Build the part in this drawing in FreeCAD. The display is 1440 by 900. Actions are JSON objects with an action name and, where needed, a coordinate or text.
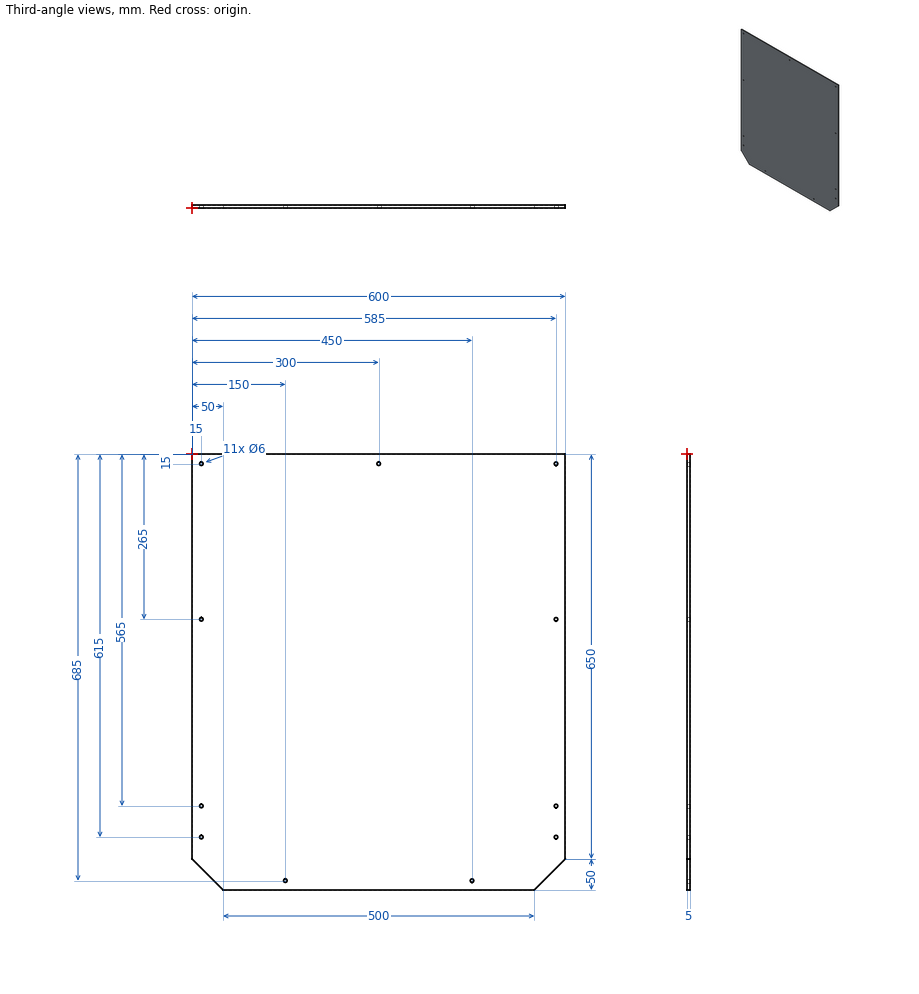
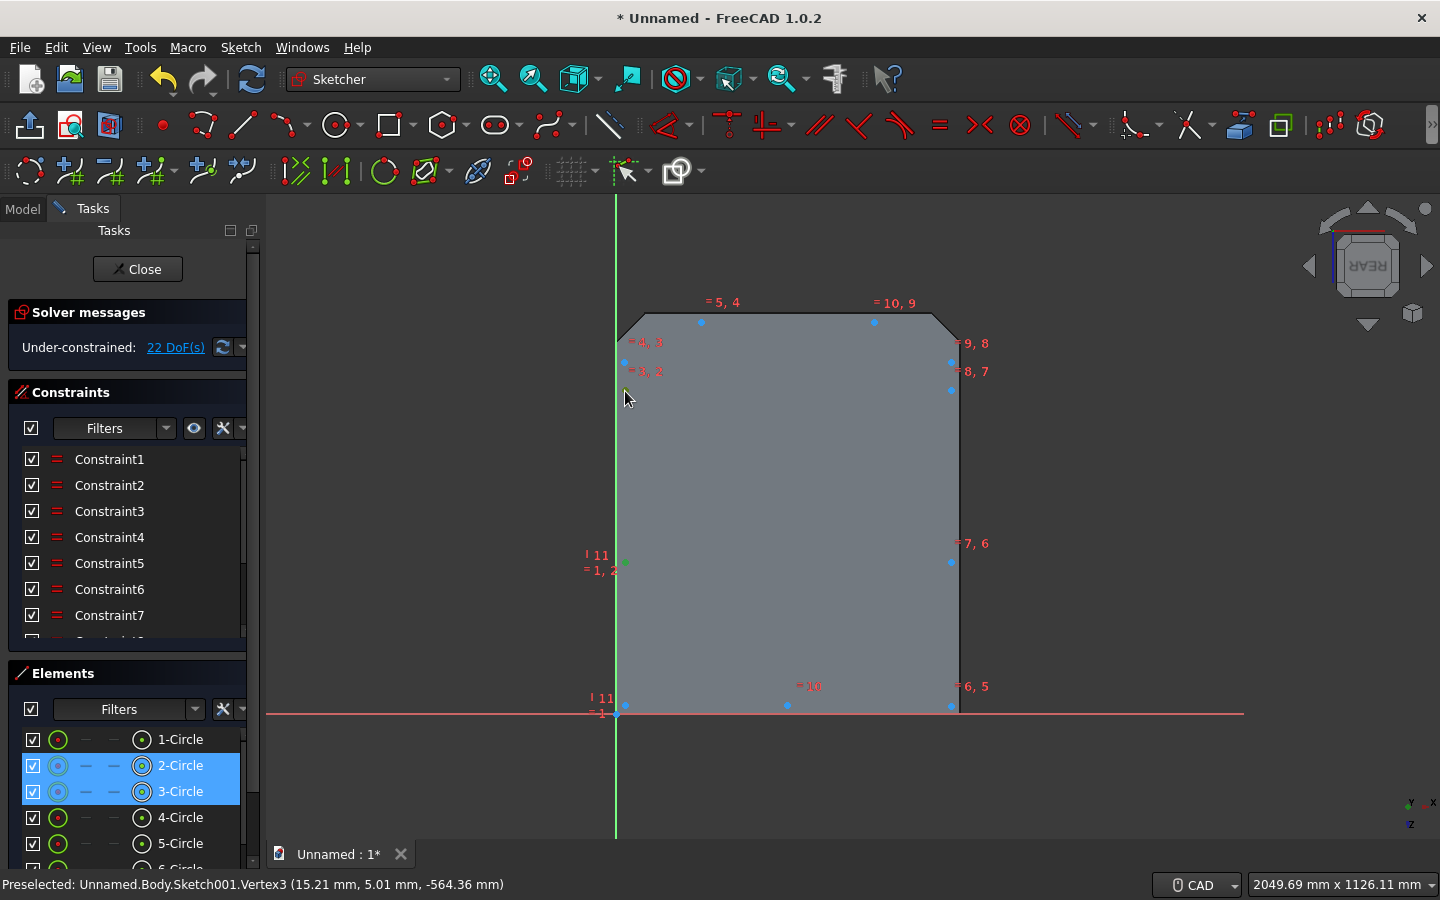
{"action": "key", "text": "v"}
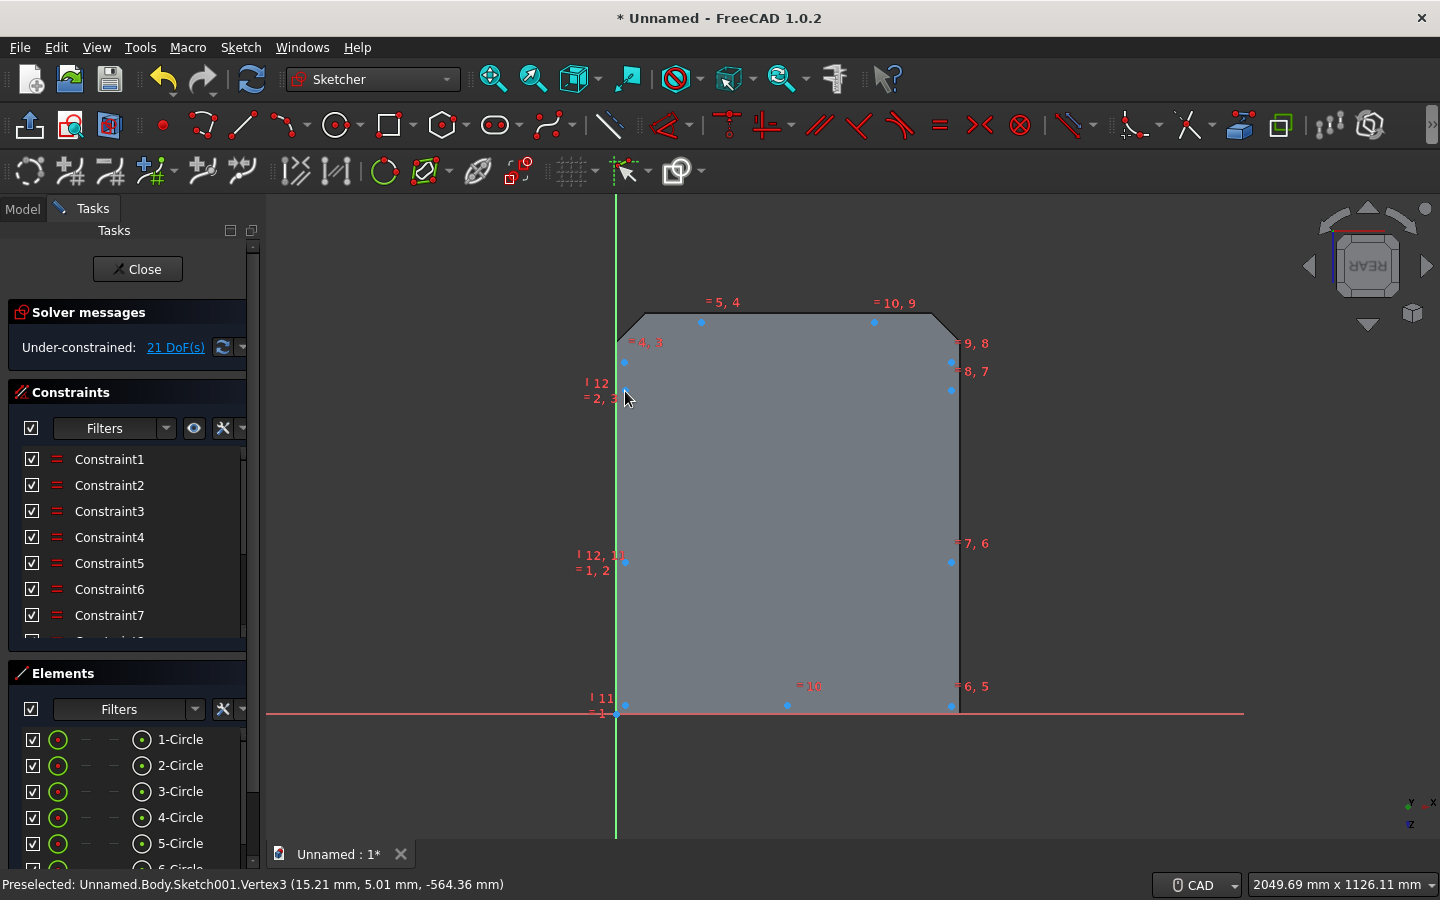
{"action": "left_click", "coordinate": [625, 391]}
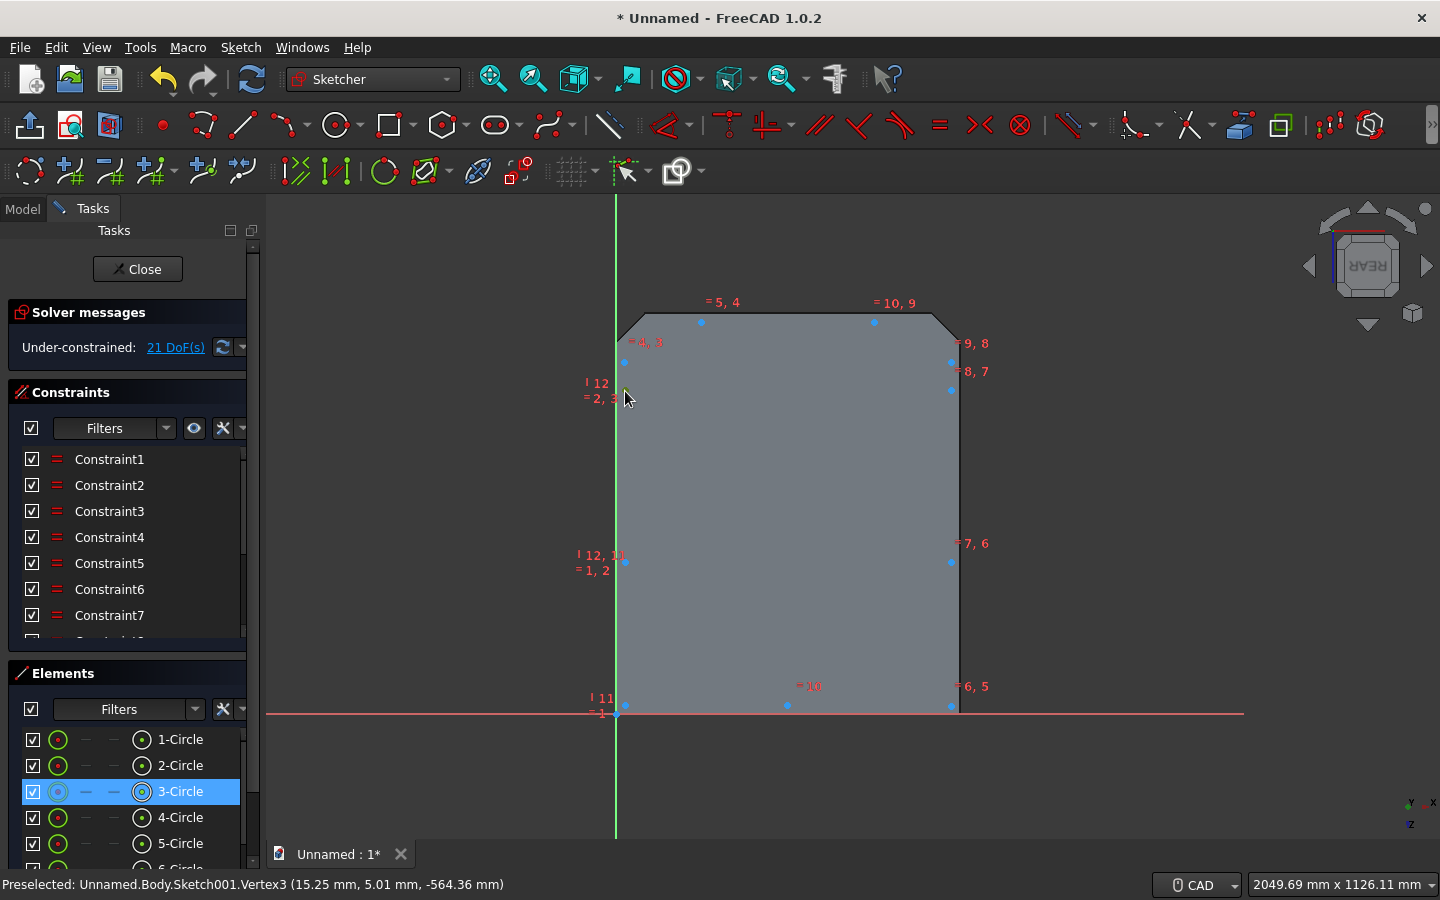
{"action": "left_click", "coordinate": [625, 362]}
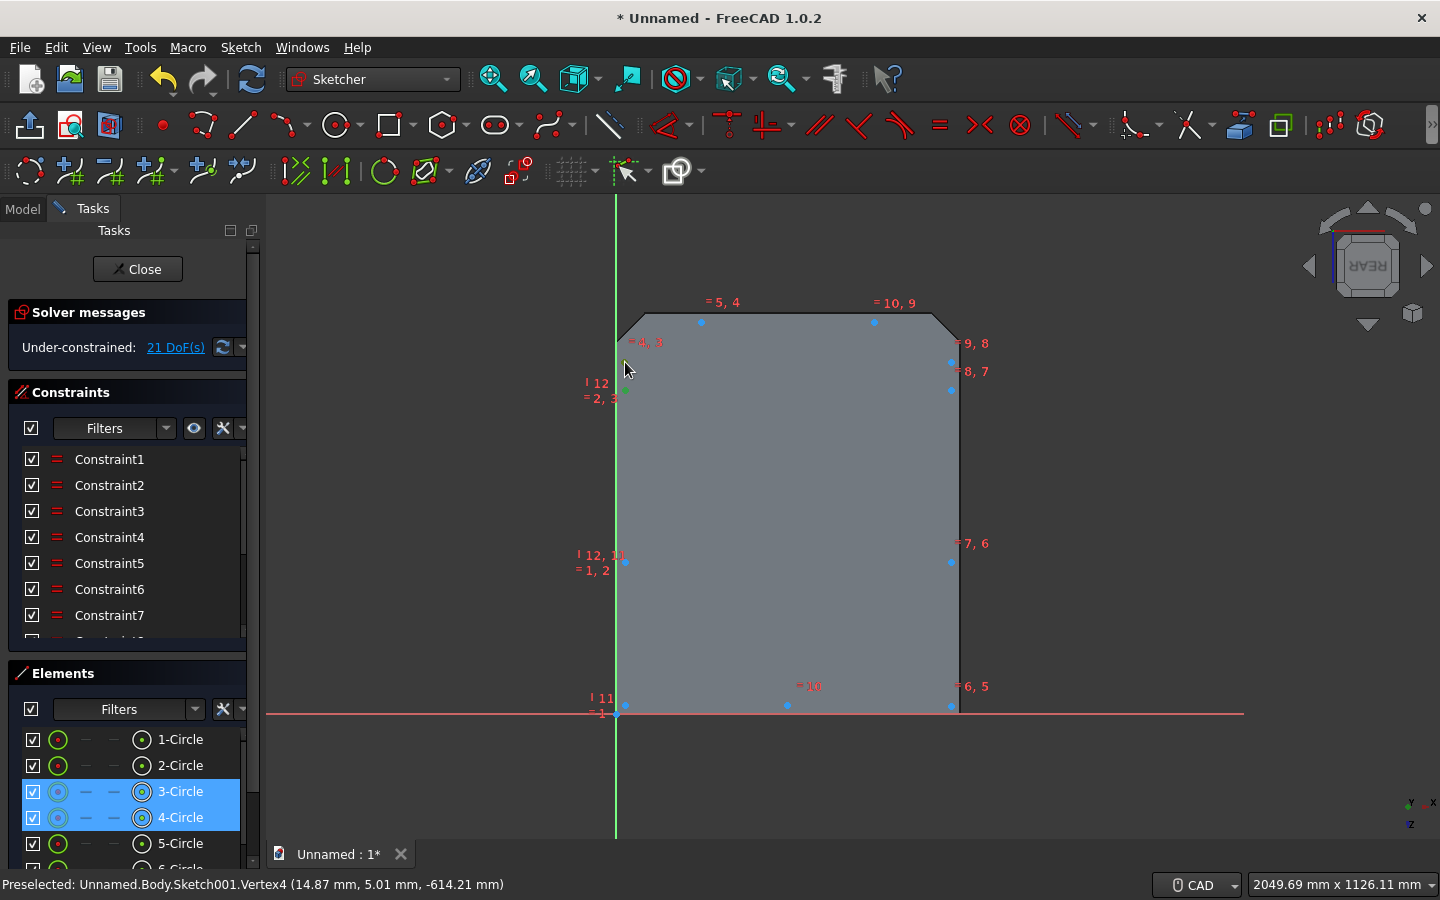
{"action": "key", "text": "v"}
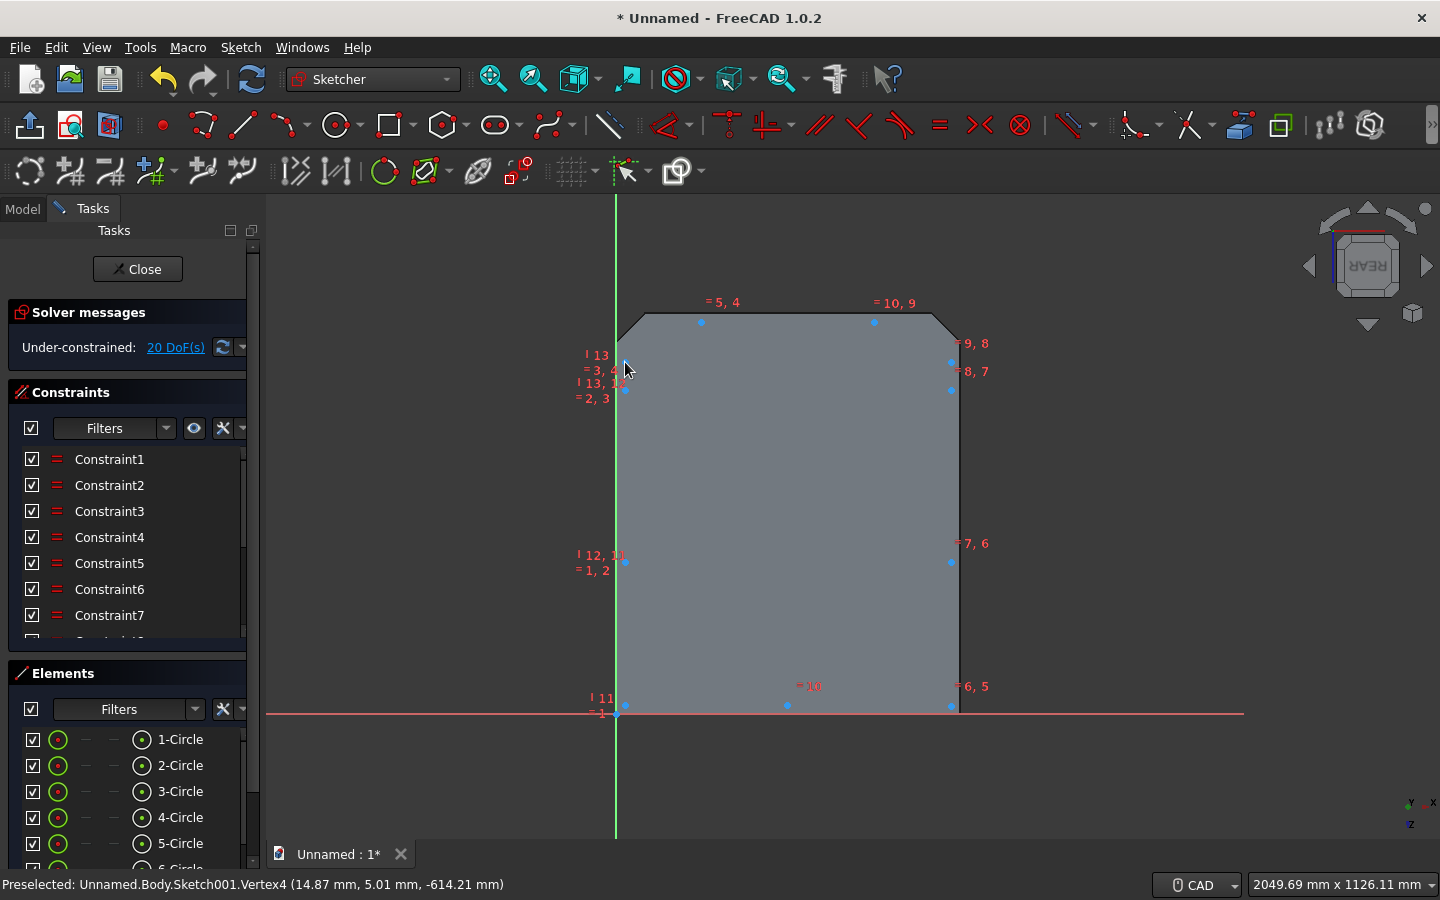
{"action": "left_click", "coordinate": [625, 706]}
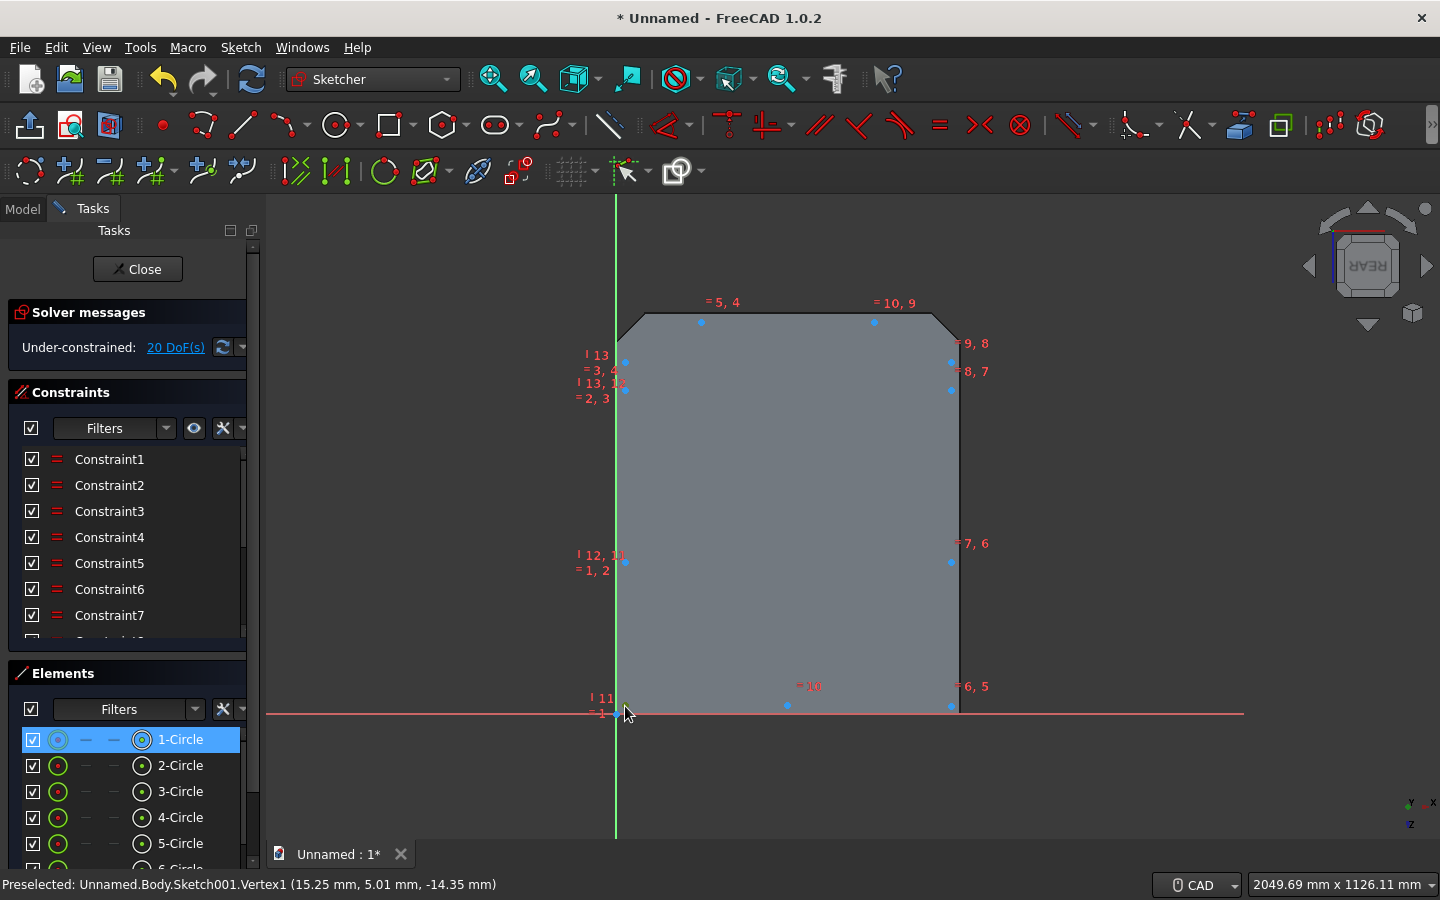
{"action": "left_click", "coordinate": [951, 706]}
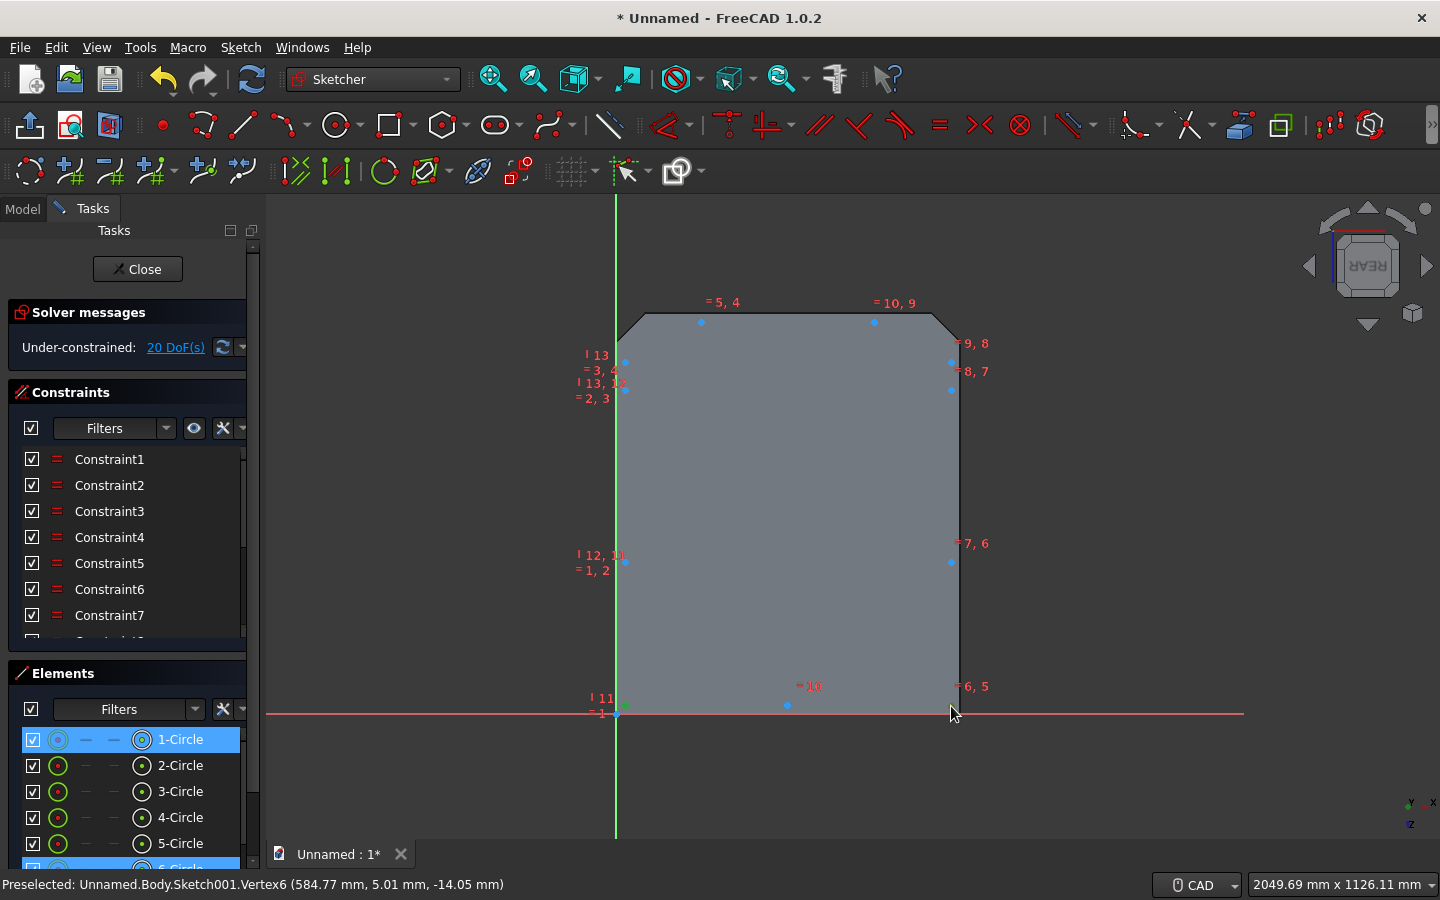
{"action": "left_click", "coordinate": [794, 126]}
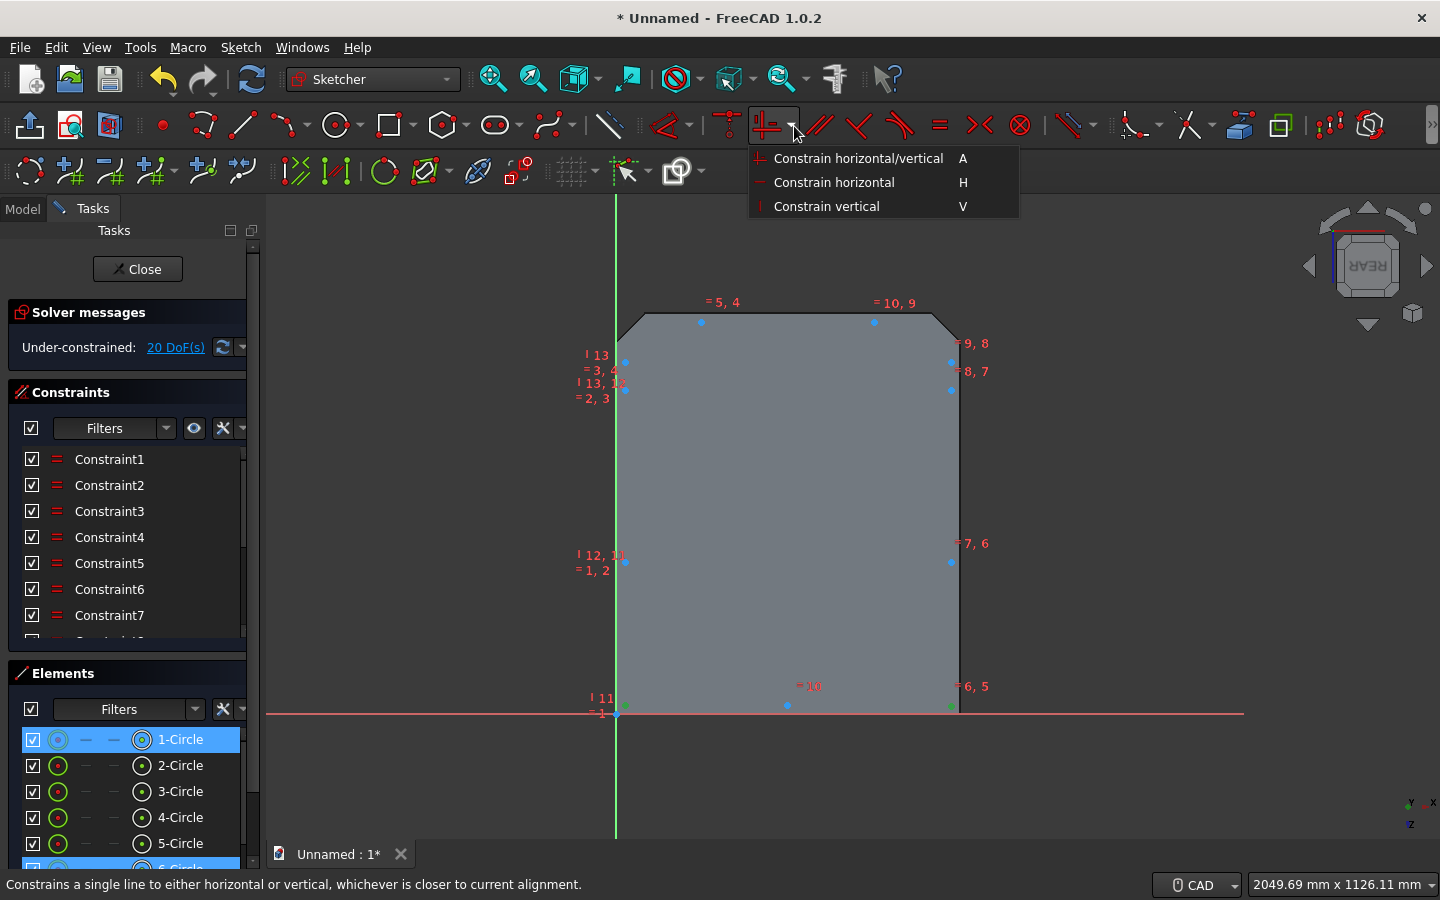
{"action": "left_click", "coordinate": [884, 182]}